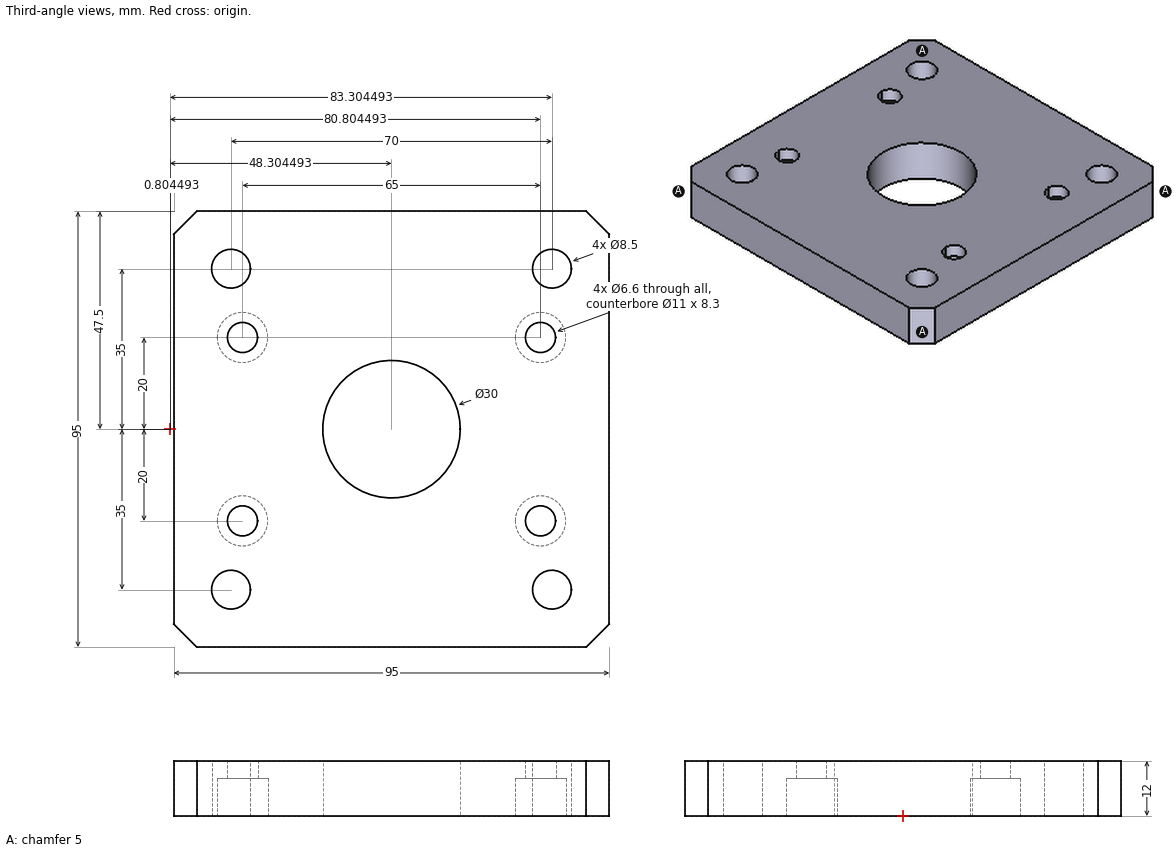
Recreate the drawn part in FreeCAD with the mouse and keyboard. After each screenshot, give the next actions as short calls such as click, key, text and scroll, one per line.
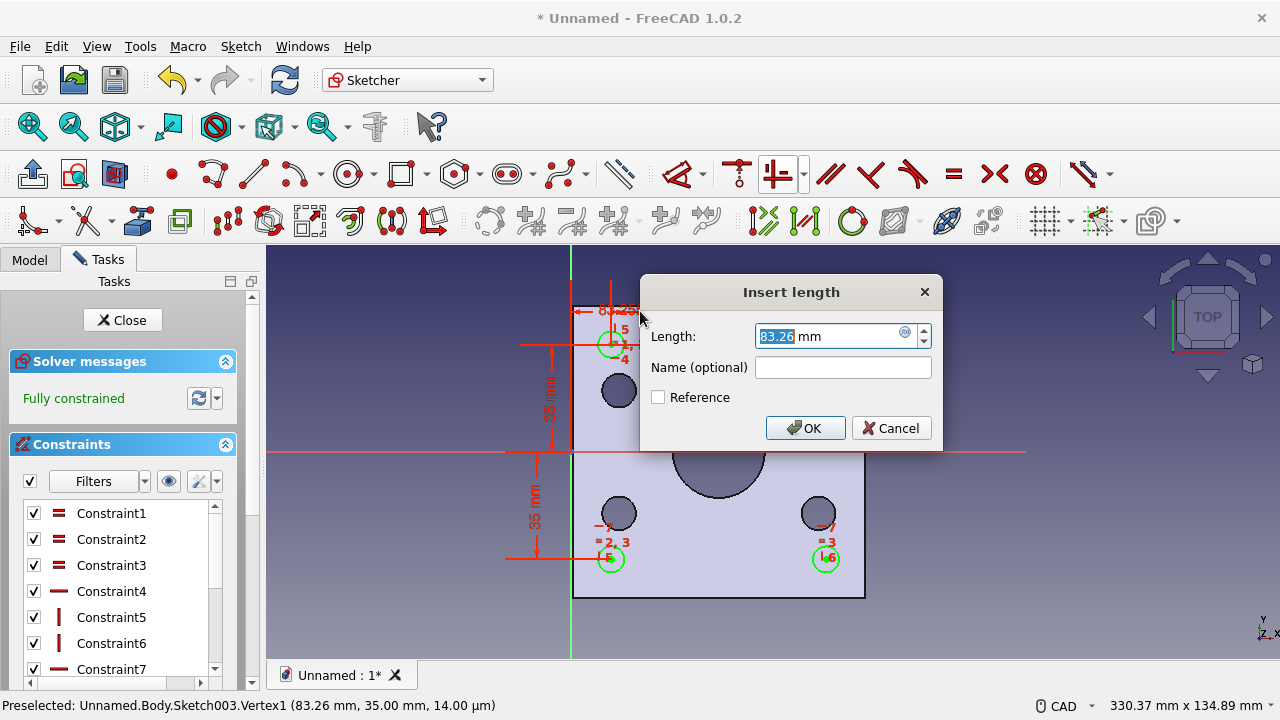
text(83.304493)
key(Return)
key(Escape)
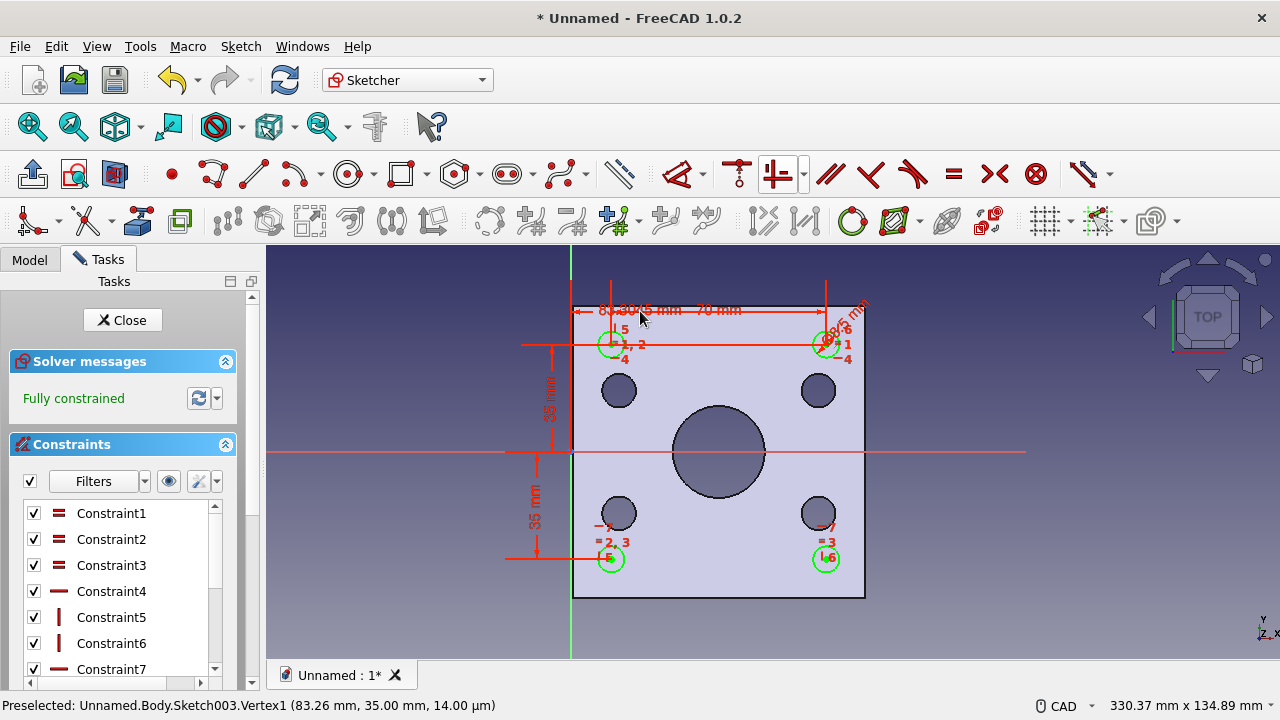
click(123, 320)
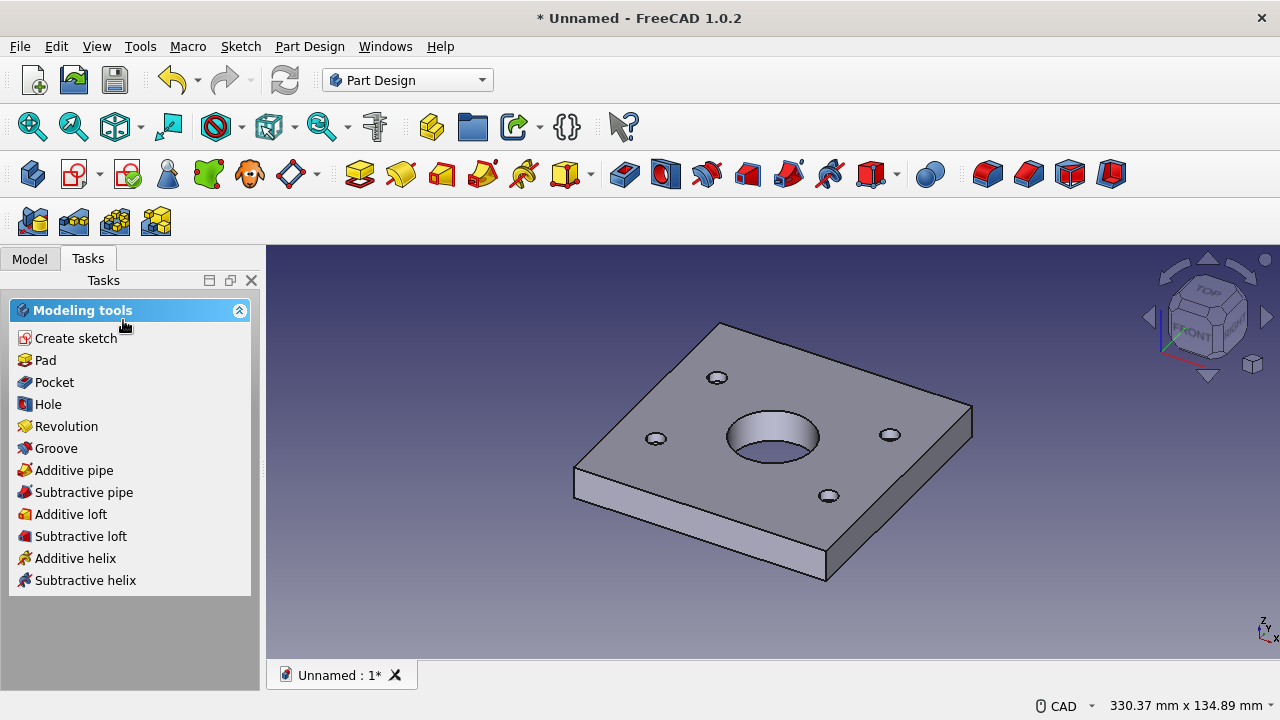
click(625, 174)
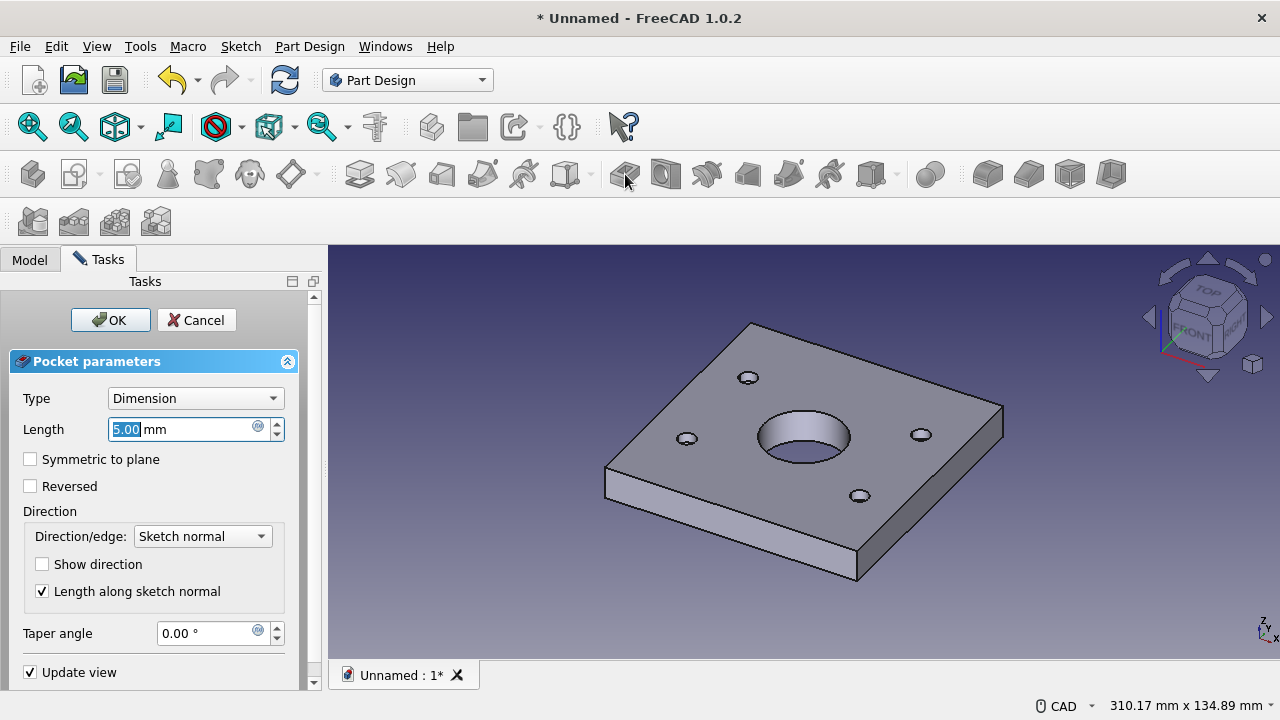
click(196, 398)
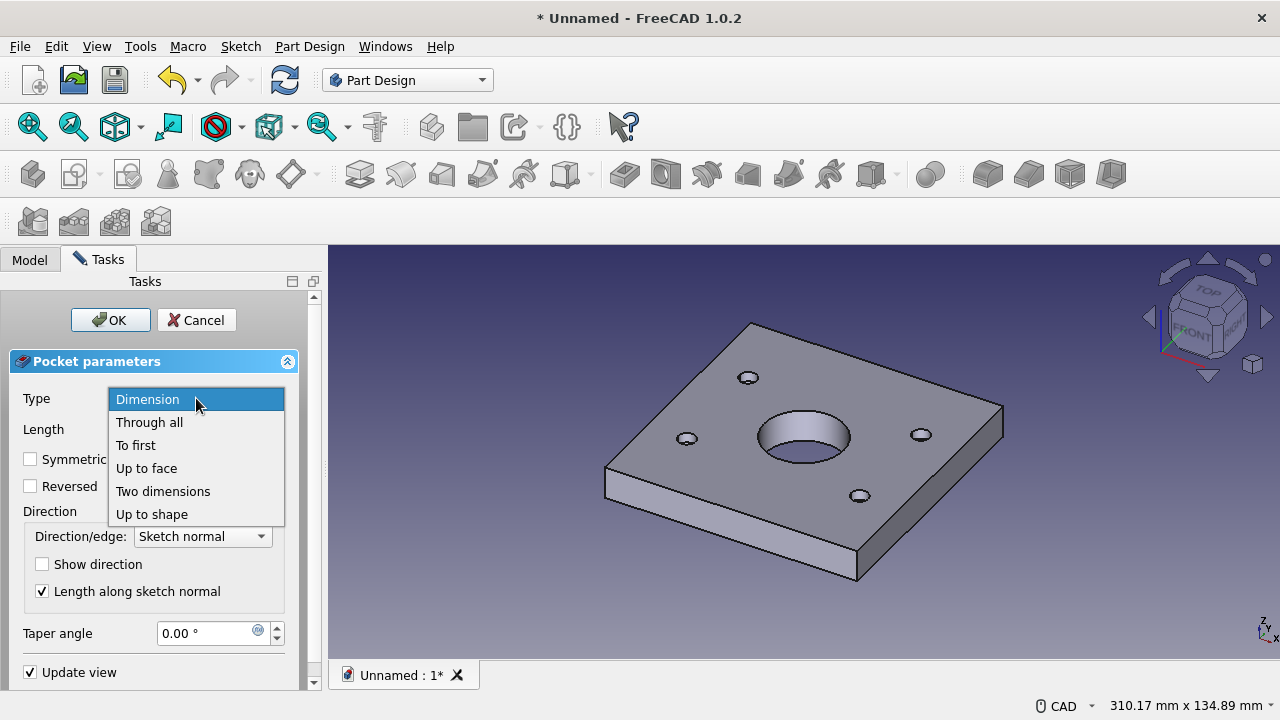
click(194, 422)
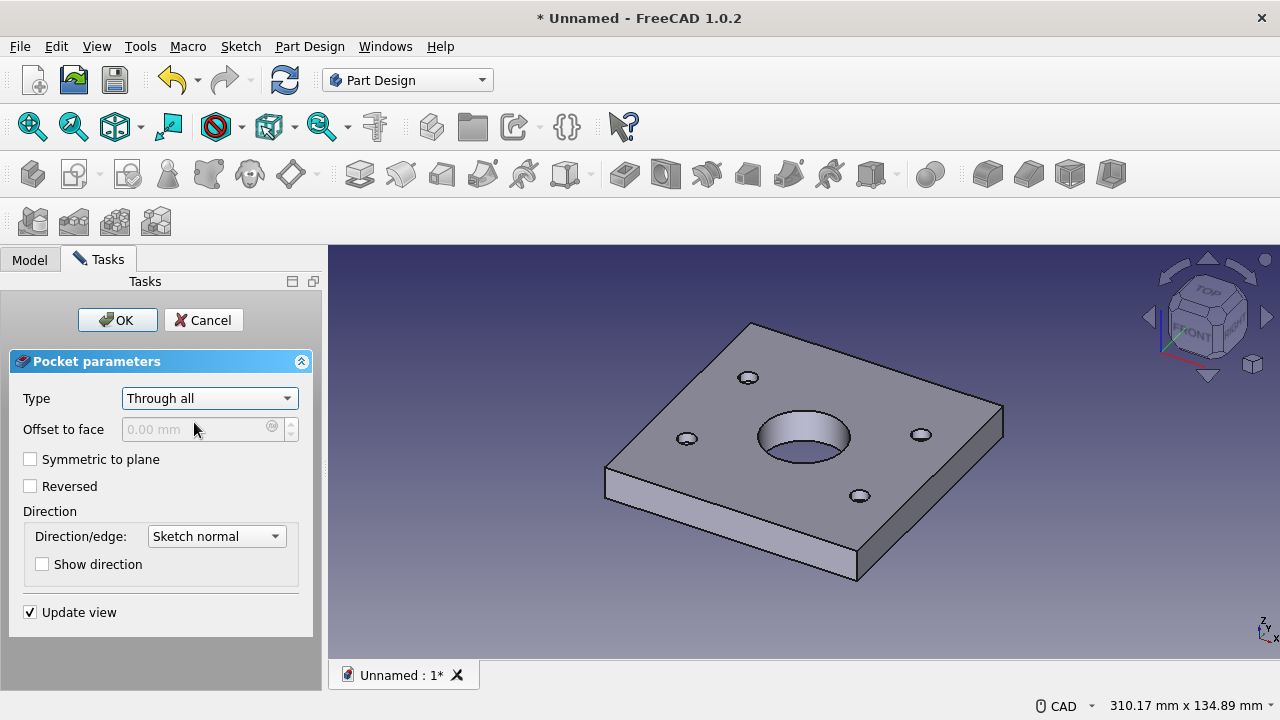
click(31, 486)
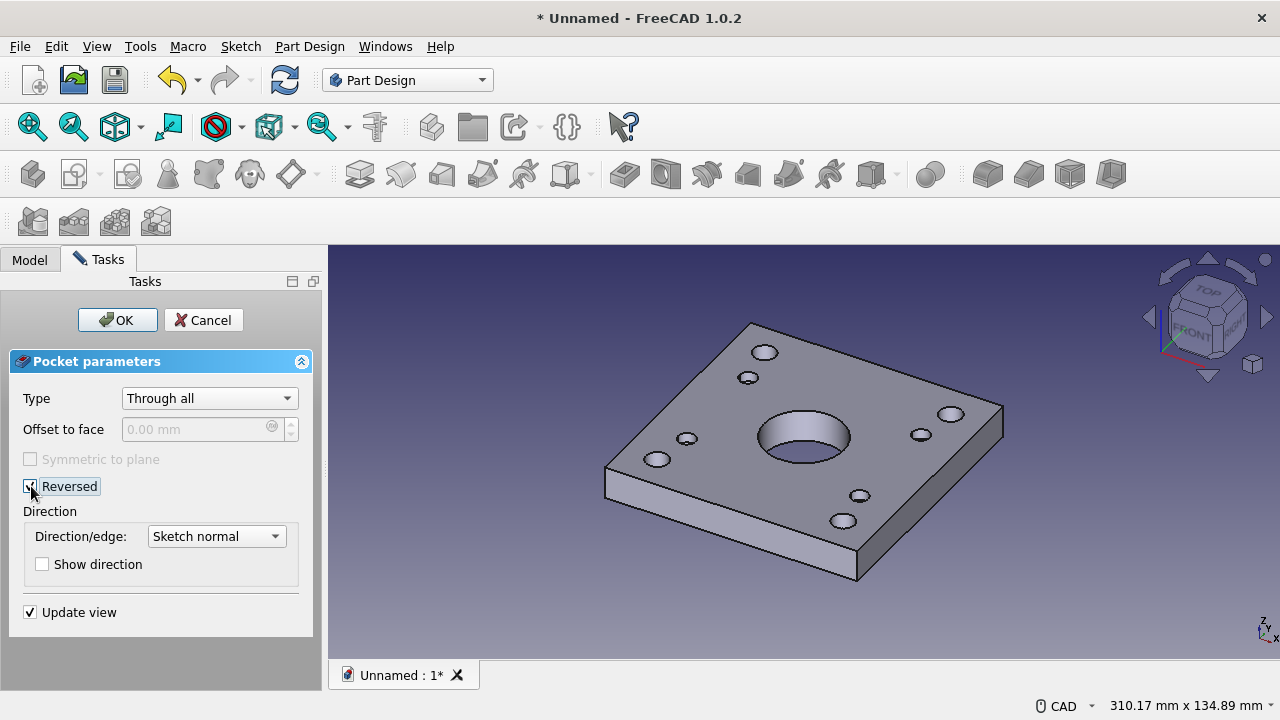
click(118, 320)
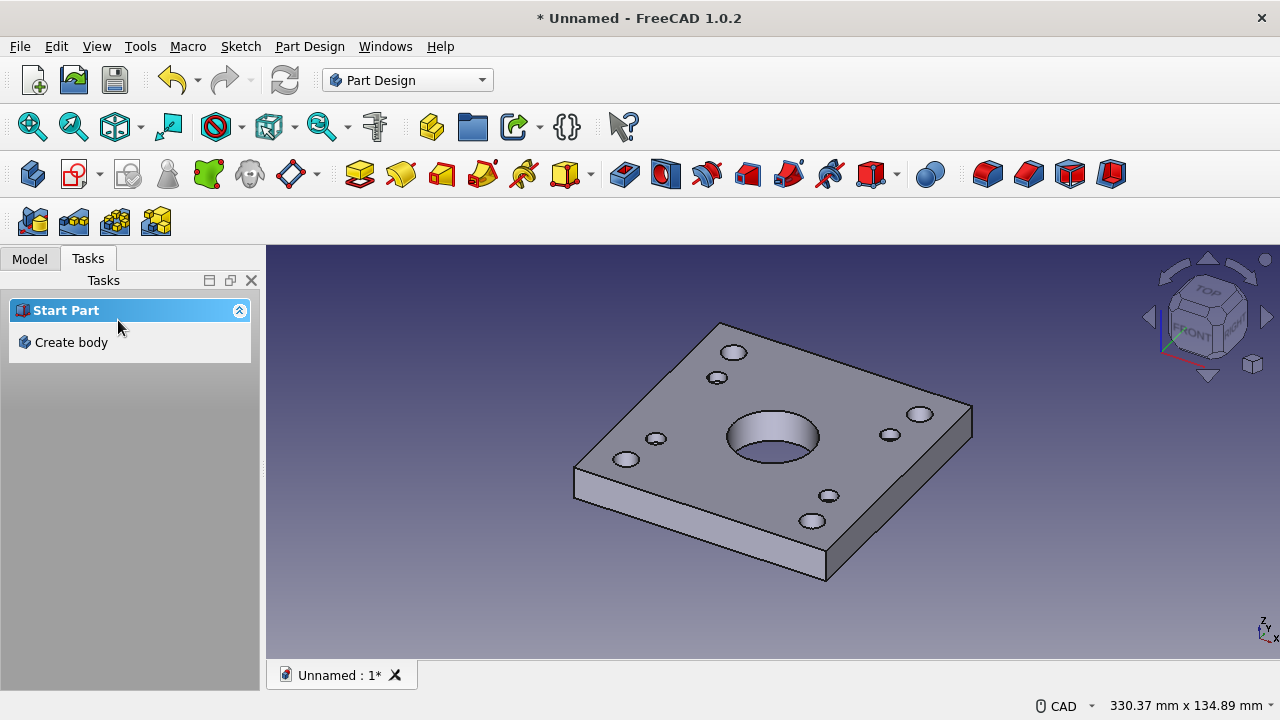
click(826, 565)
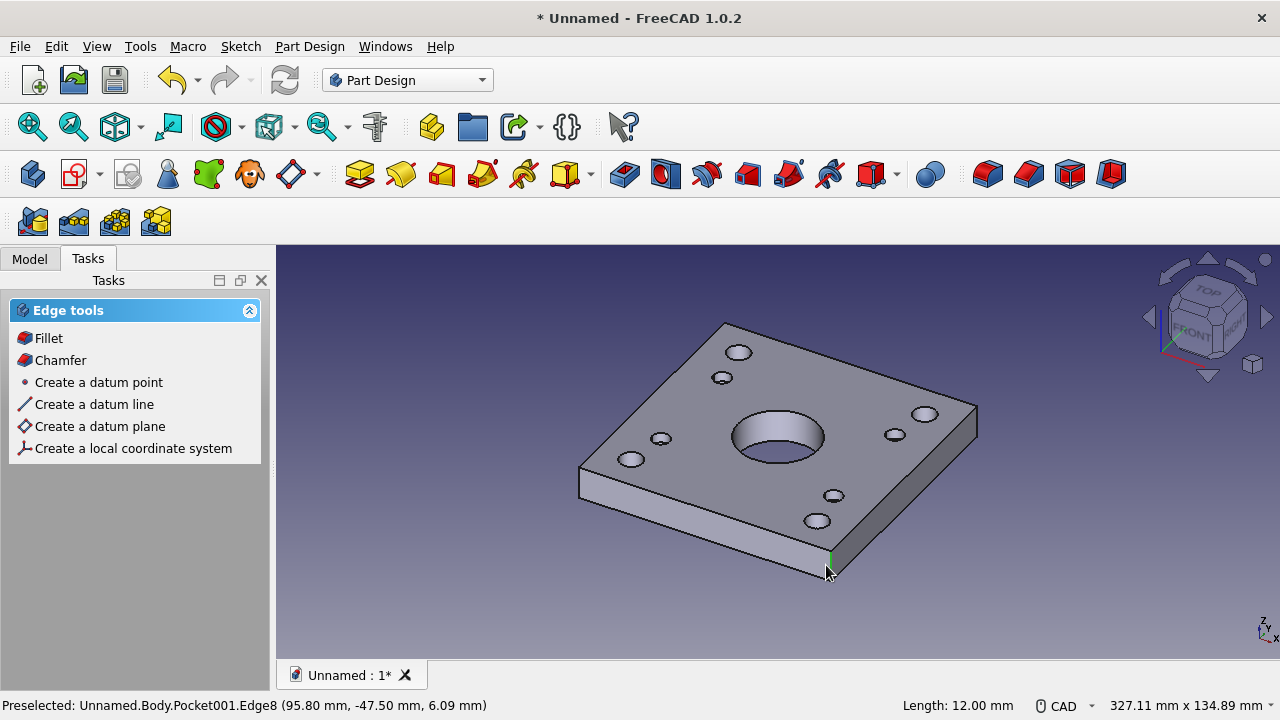
key(0)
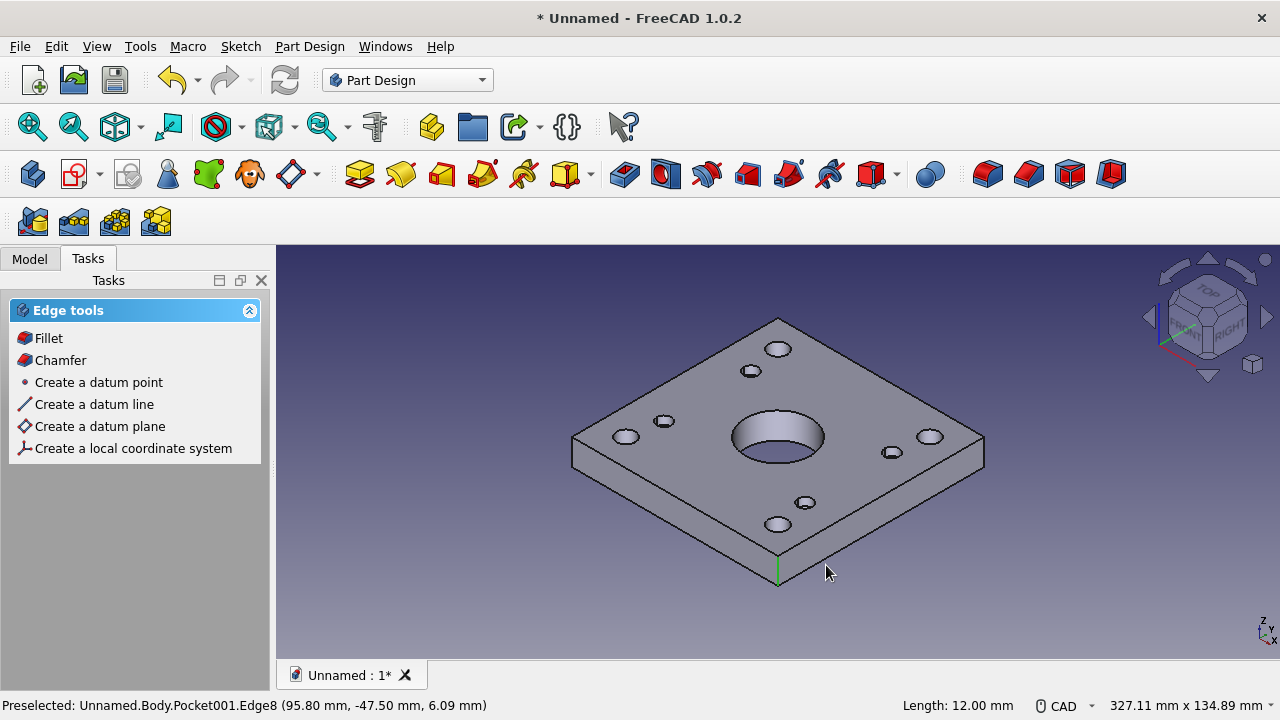
key(2)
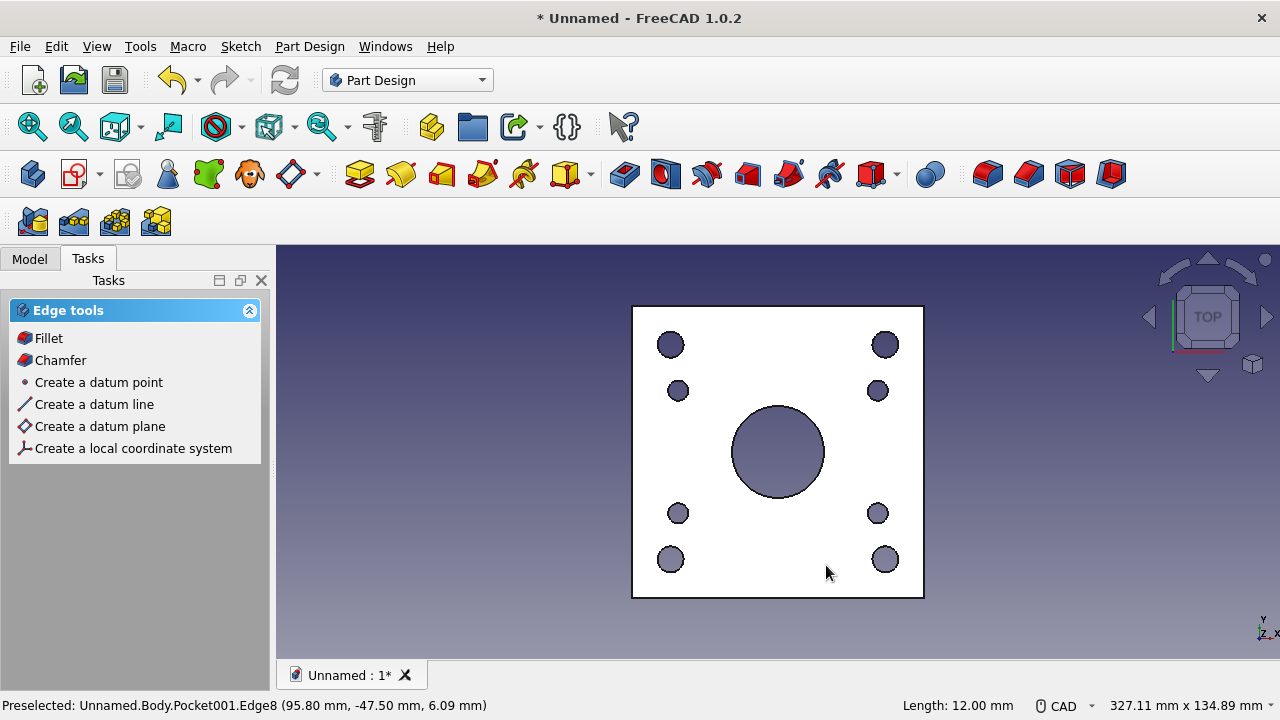
key(1)